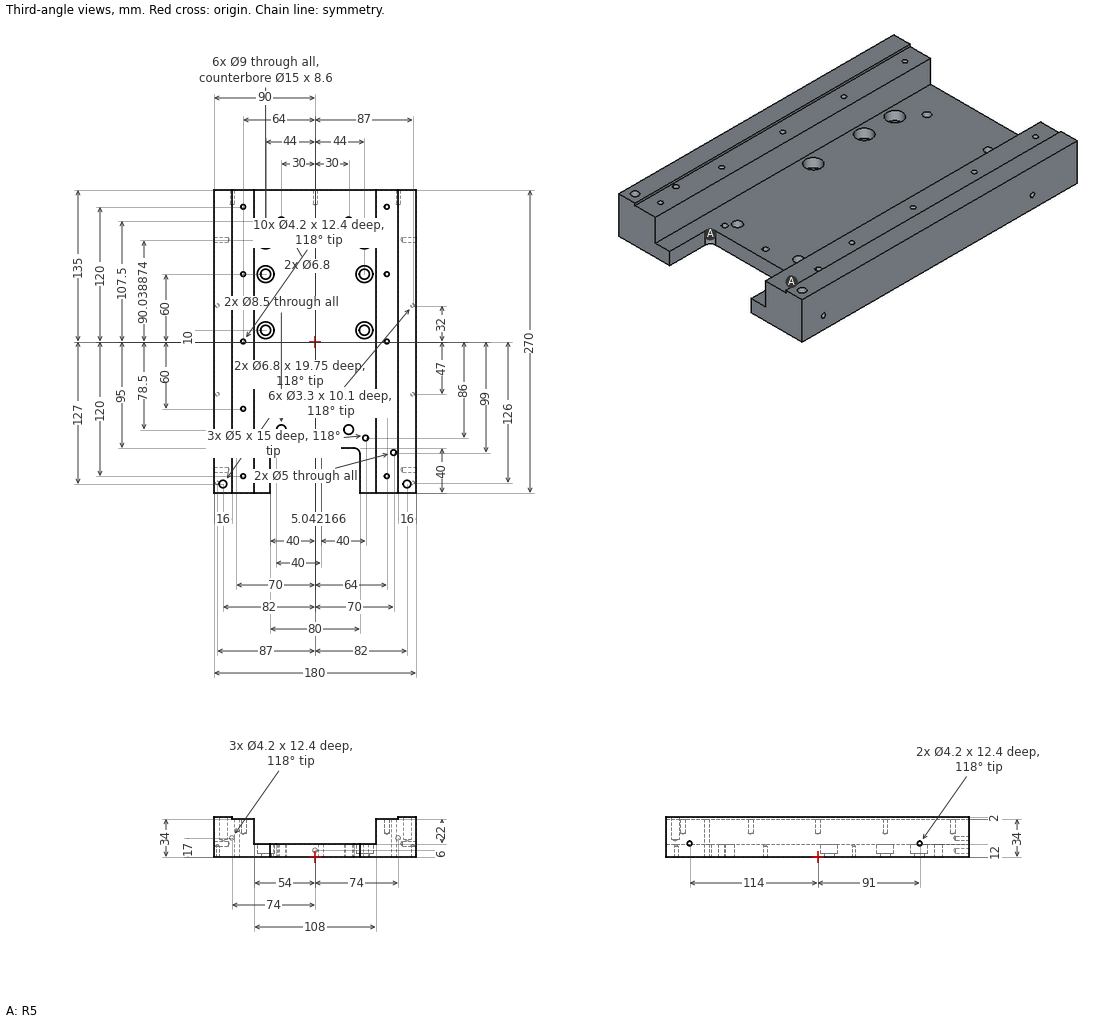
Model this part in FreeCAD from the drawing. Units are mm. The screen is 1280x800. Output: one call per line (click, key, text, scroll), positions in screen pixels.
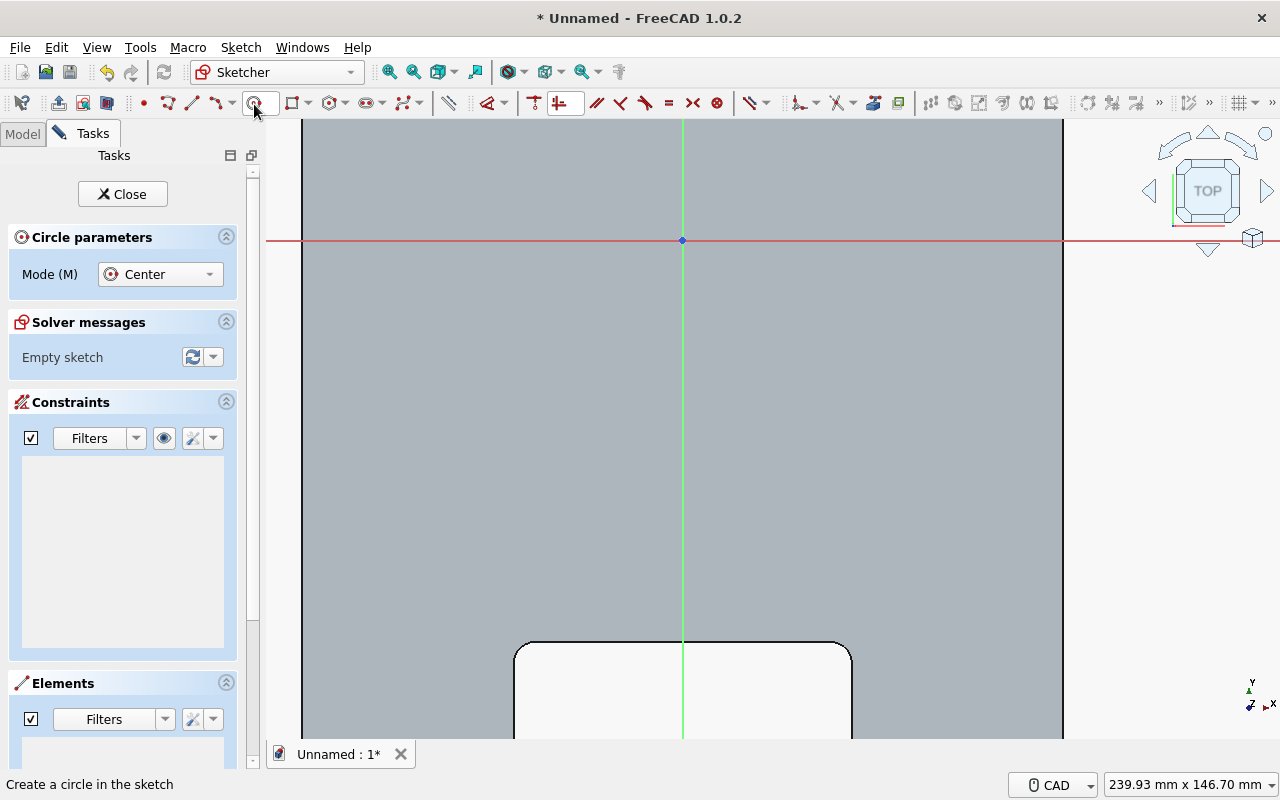
scroll(873, 604, up, 4)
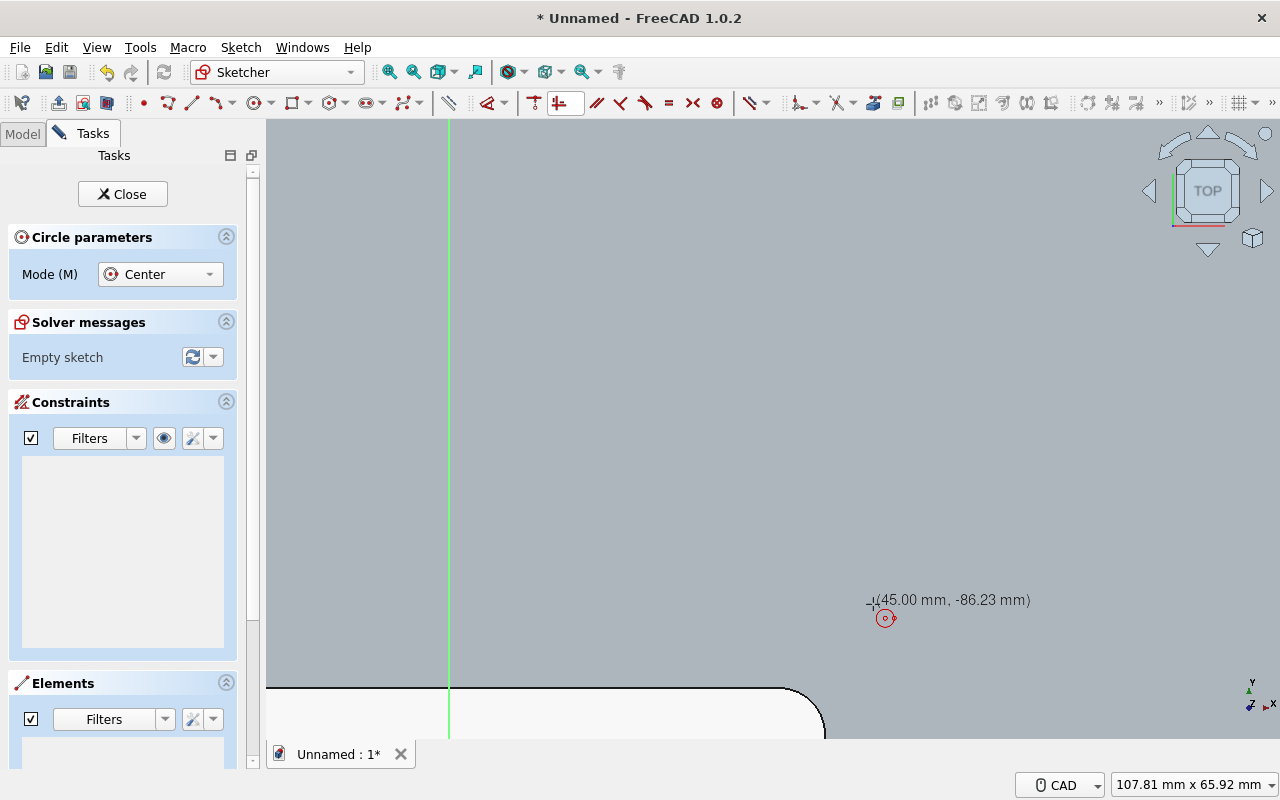
click(873, 603)
move(889, 586)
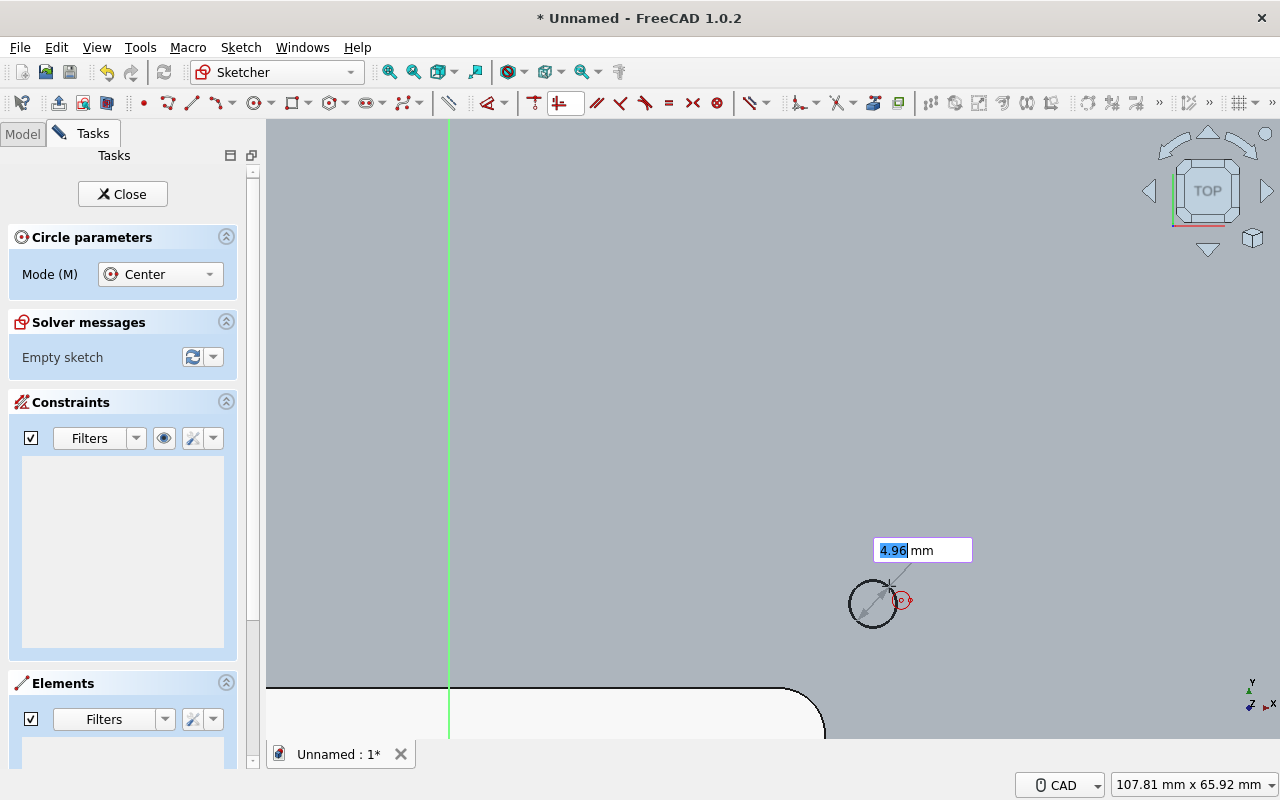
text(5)
key(Return)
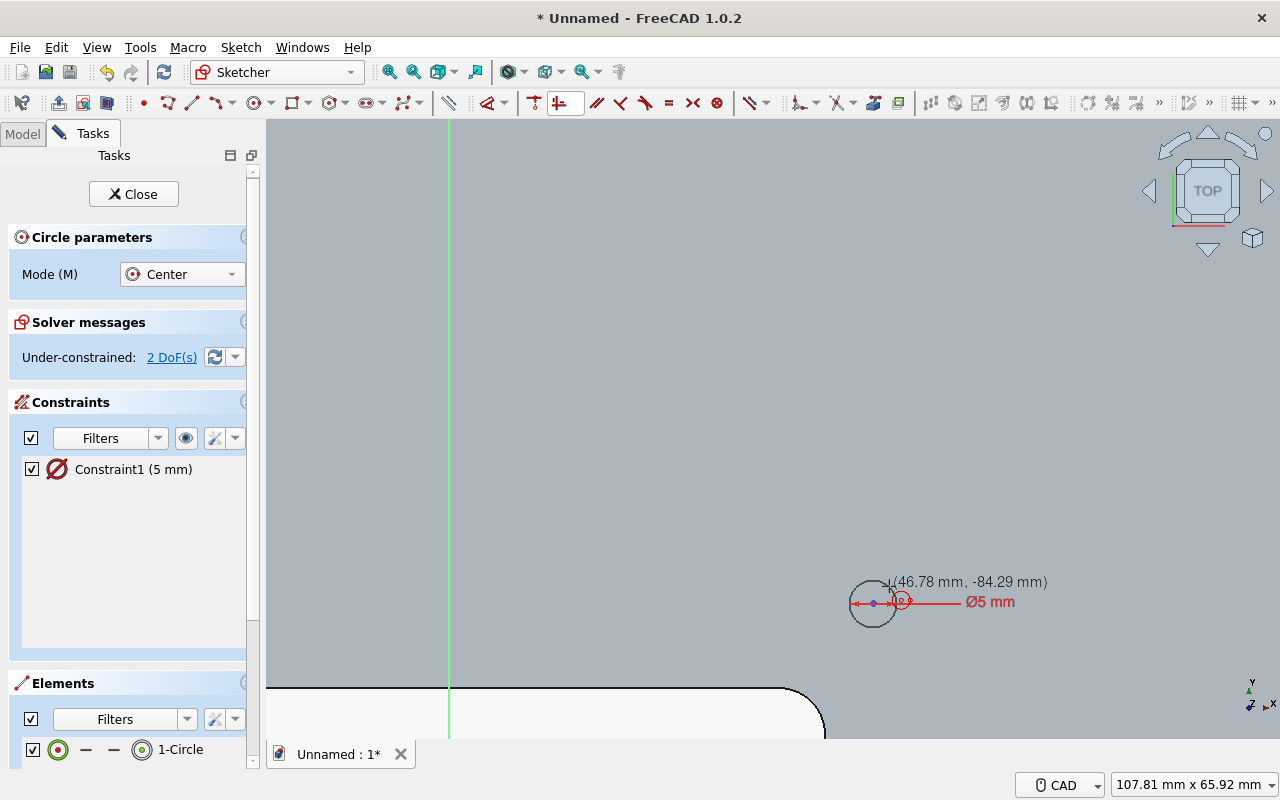
click(496, 603)
move(513, 586)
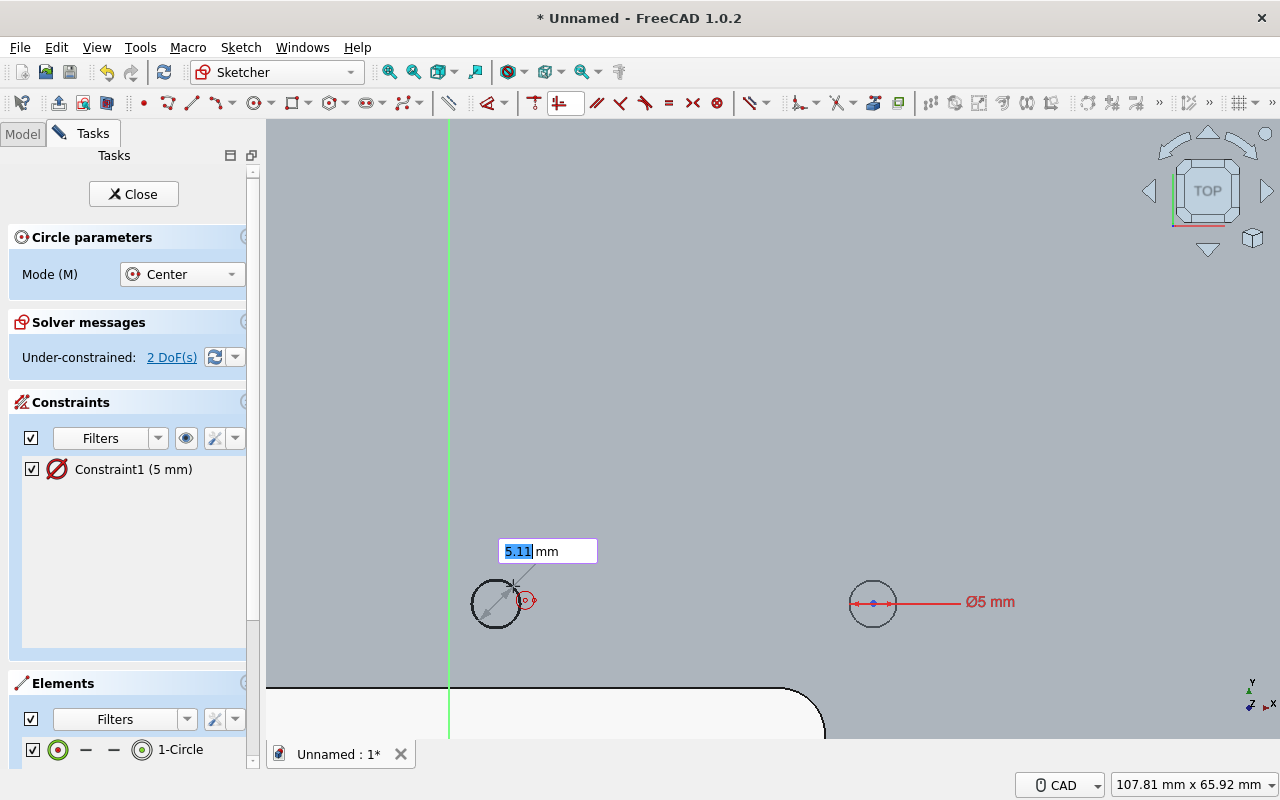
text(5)
key(Return)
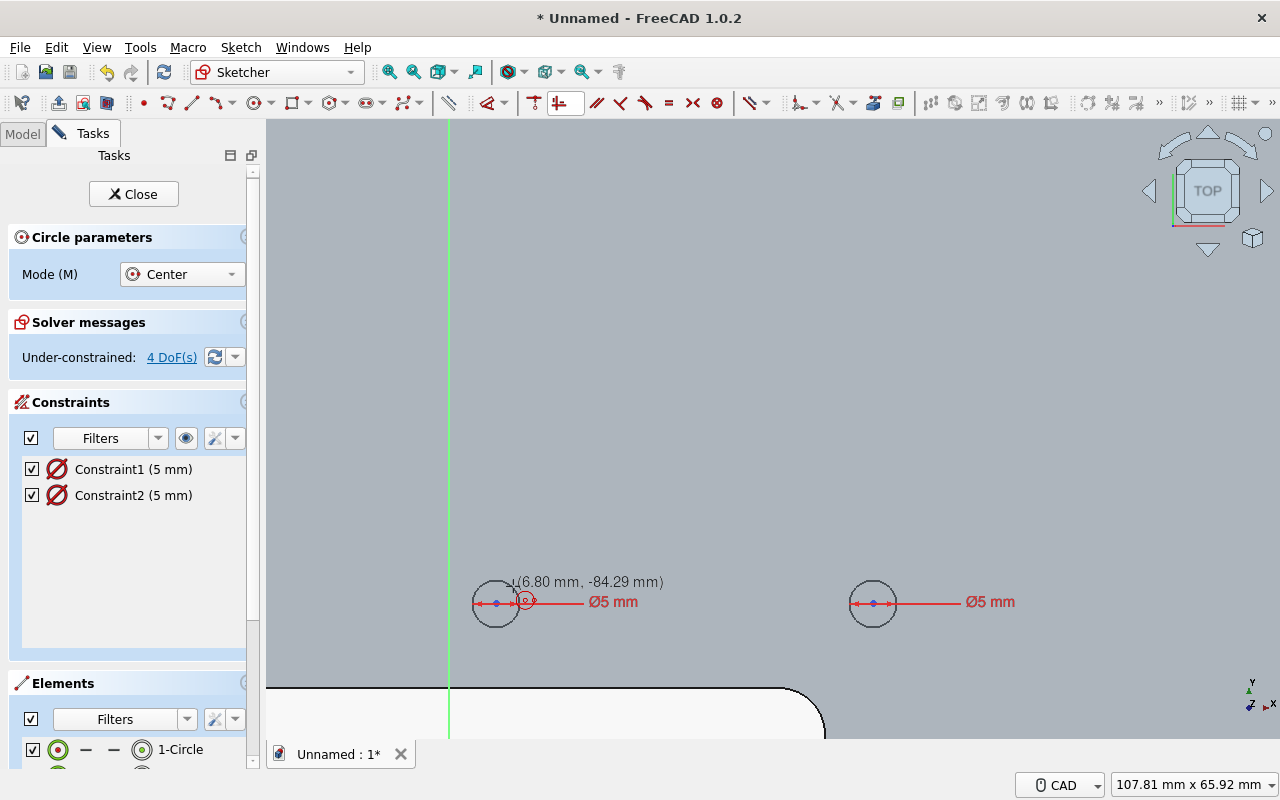
scroll(874, 607, down, 4)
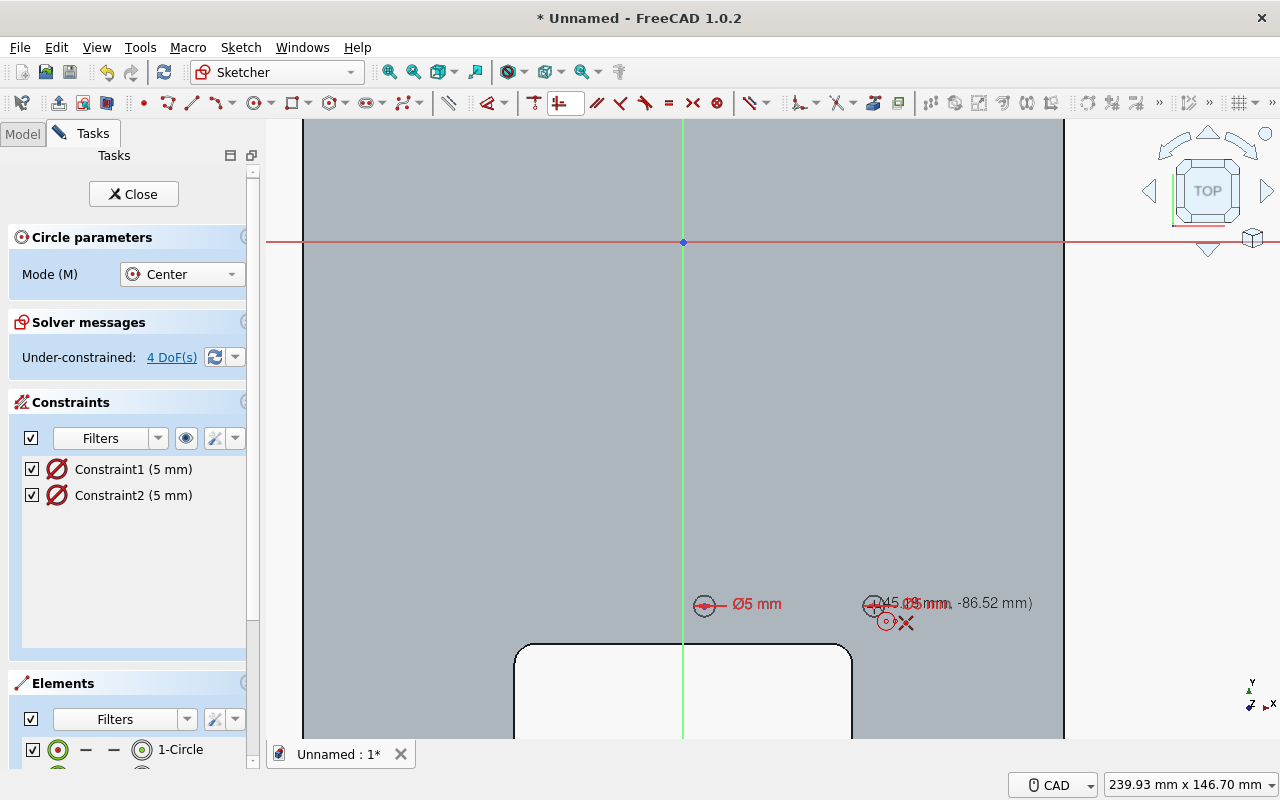
scroll(536, 606, up, 4)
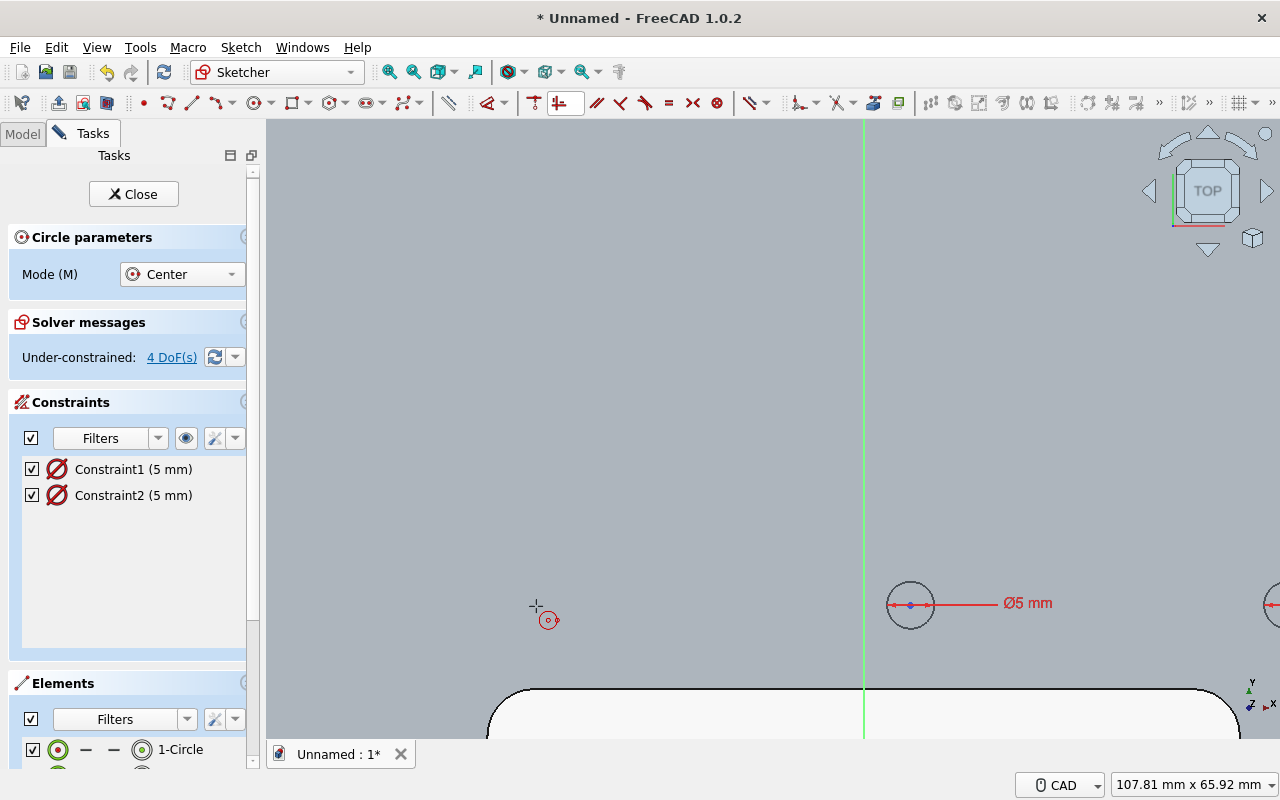
click(535, 604)
move(552, 588)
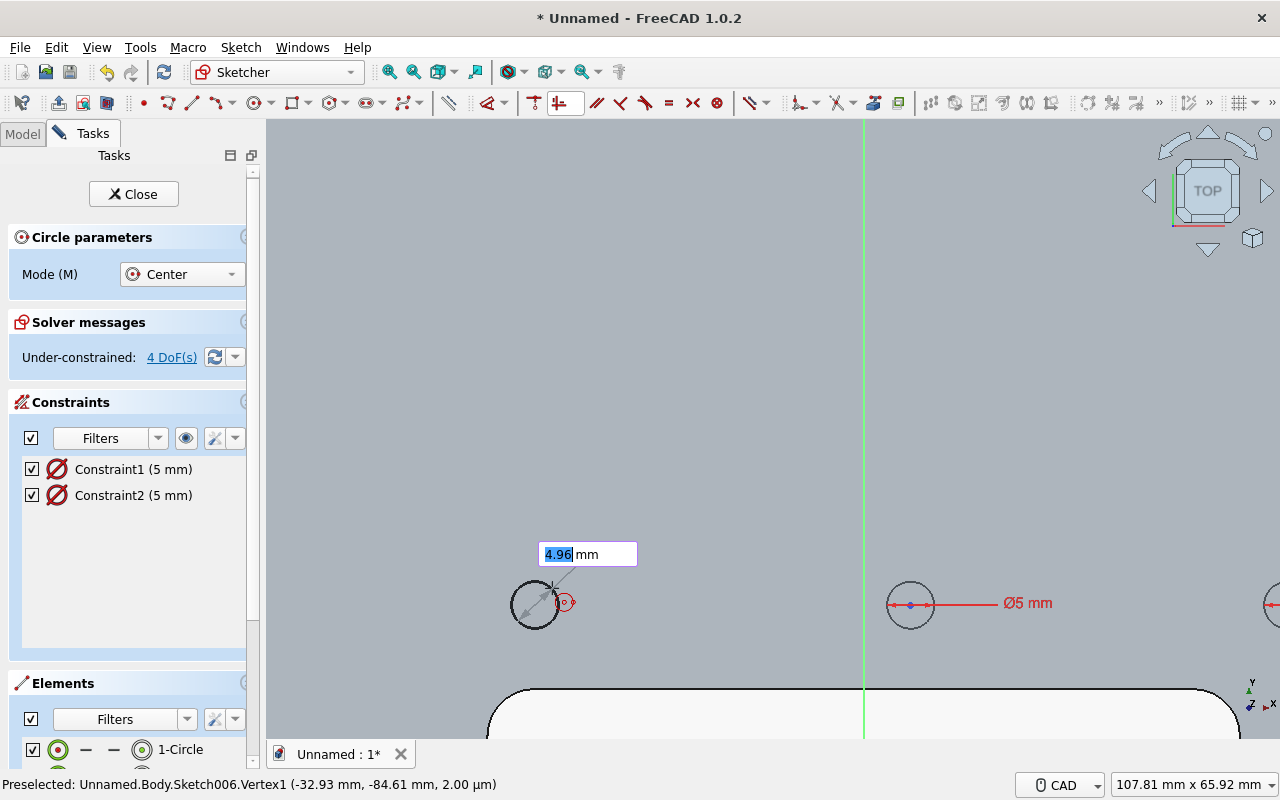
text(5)
key(Return)
key(Escape)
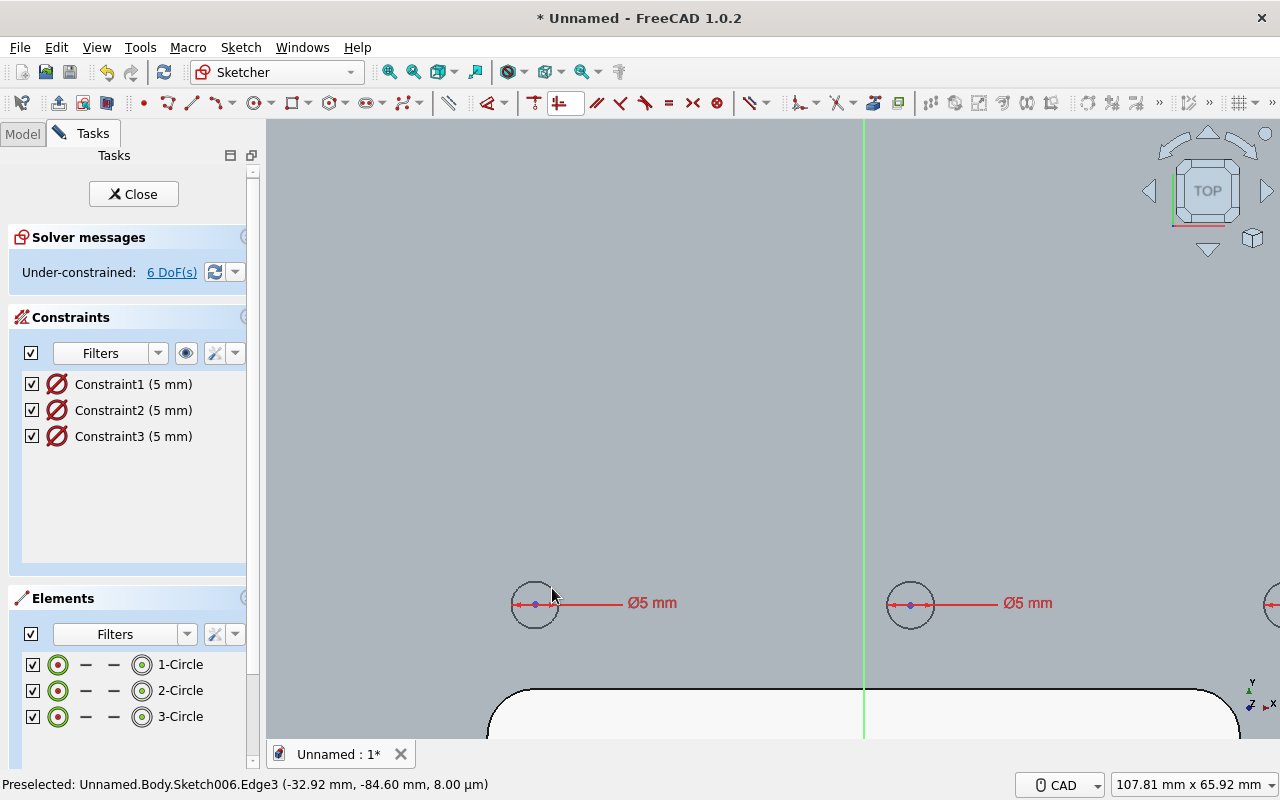
scroll(536, 606, down, 4)